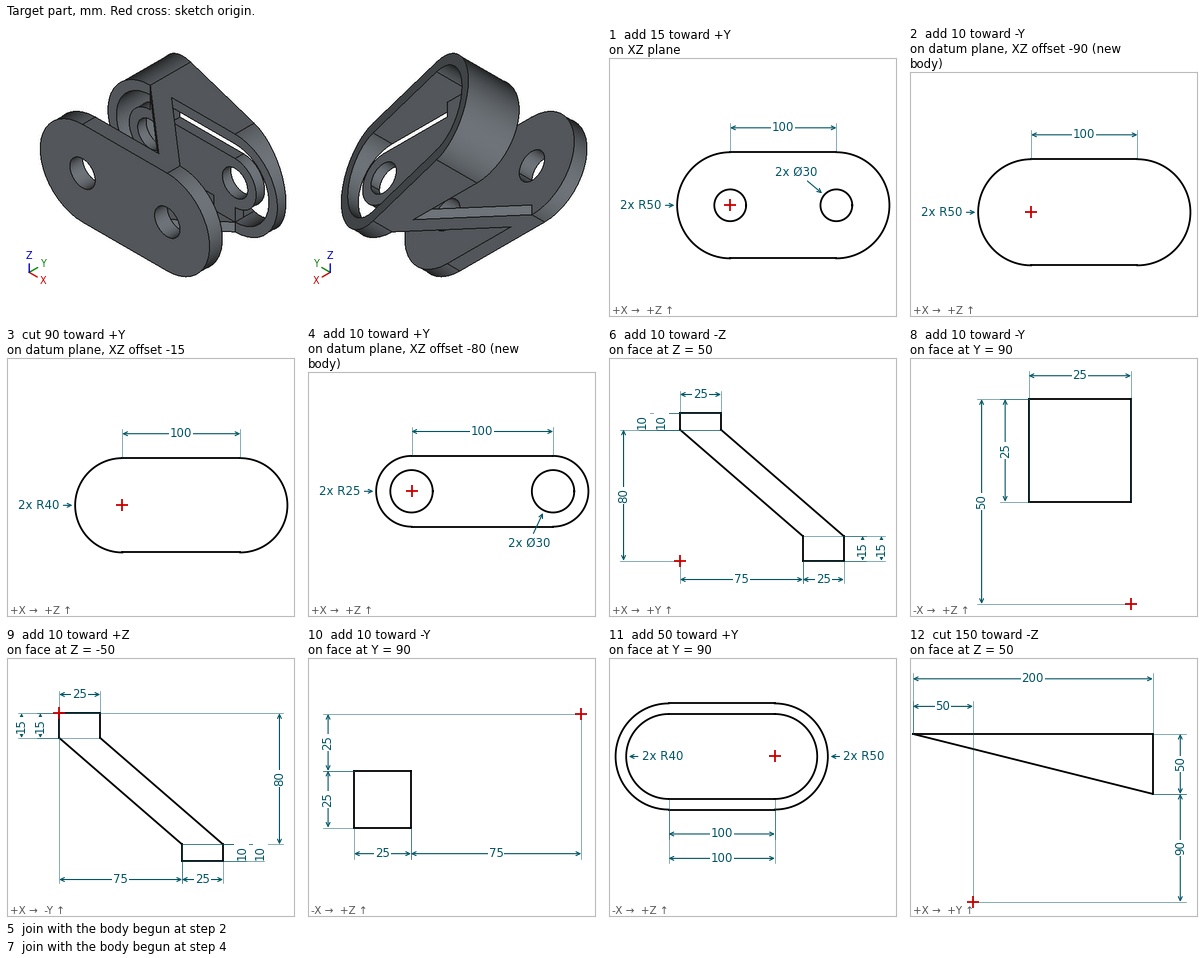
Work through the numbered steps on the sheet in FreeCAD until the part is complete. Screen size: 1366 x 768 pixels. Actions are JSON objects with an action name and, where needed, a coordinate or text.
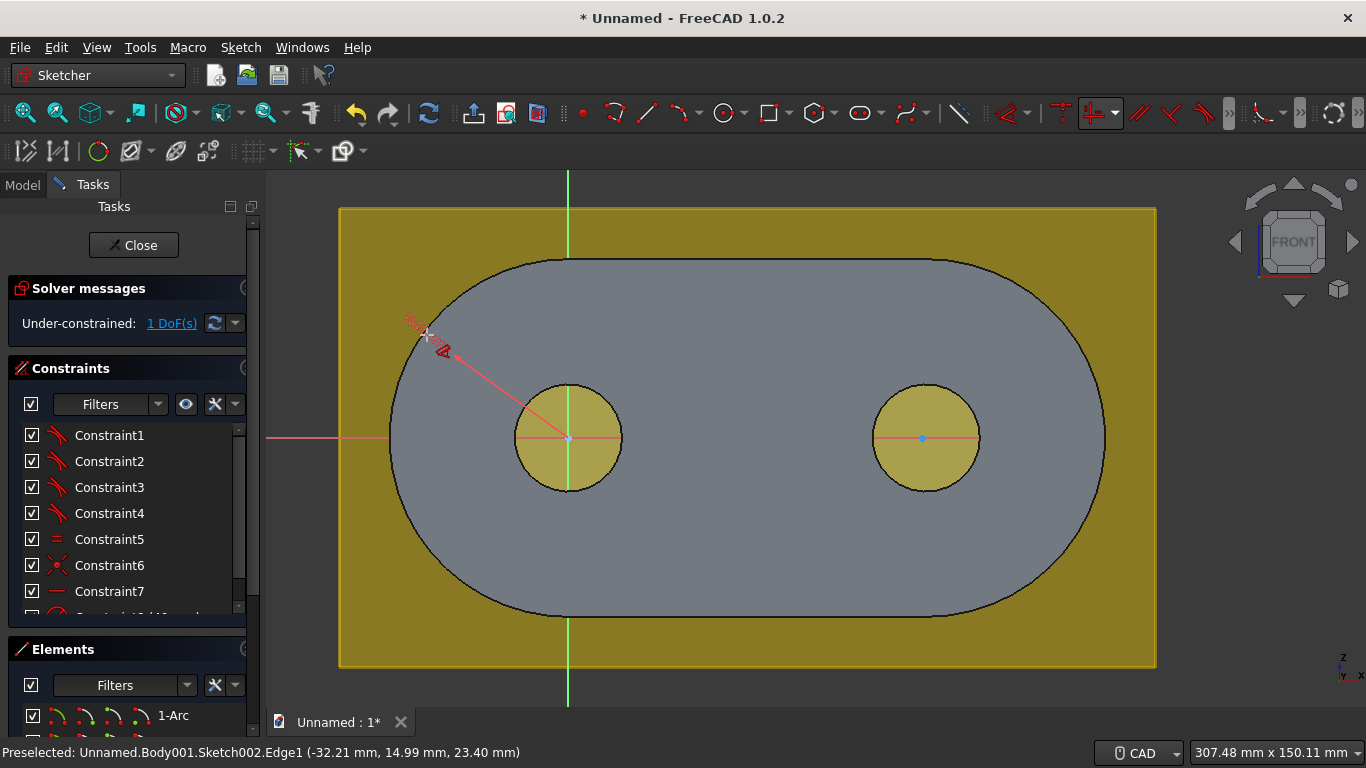
{"action": "left_click", "coordinate": [675, 295]}
{"action": "left_click", "coordinate": [746, 261]}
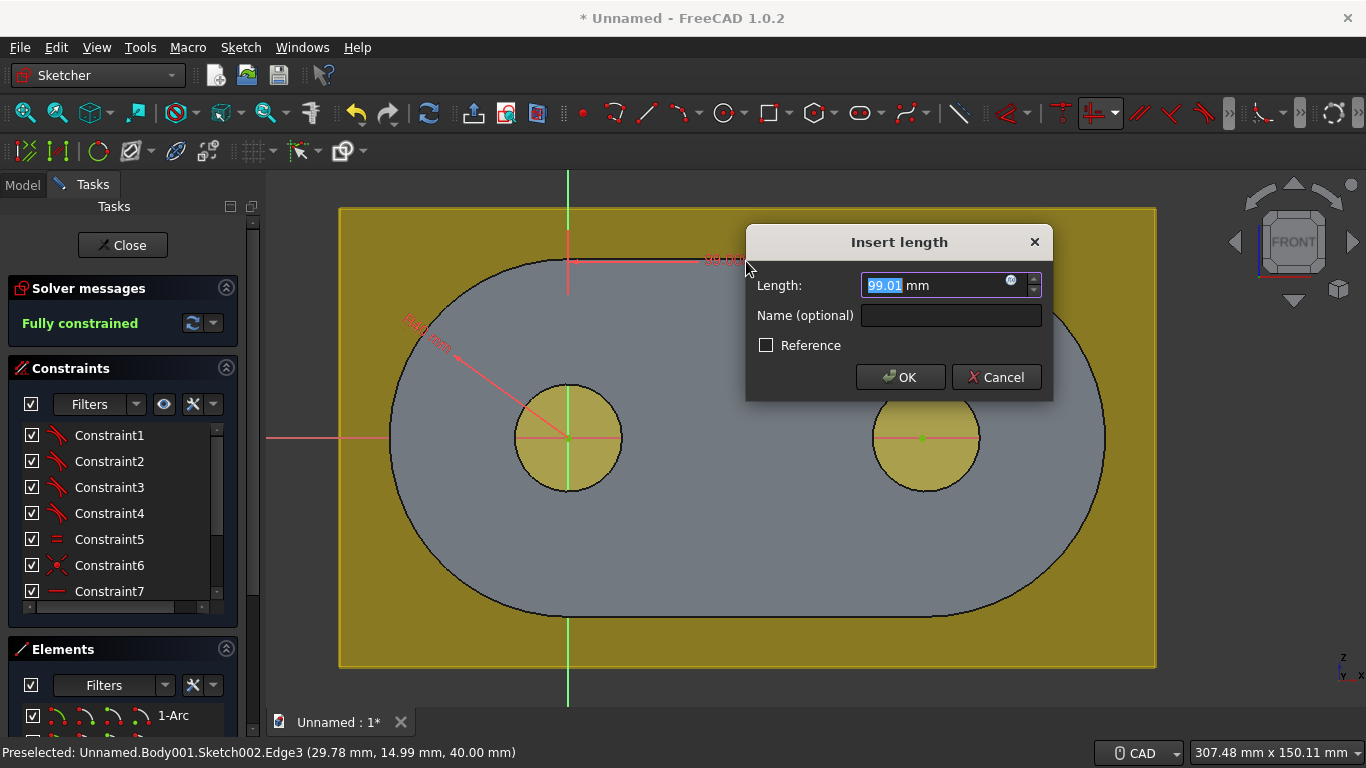
{"action": "type", "text": "100"}
{"action": "key", "text": "Return"}
{"action": "key", "text": "Escape"}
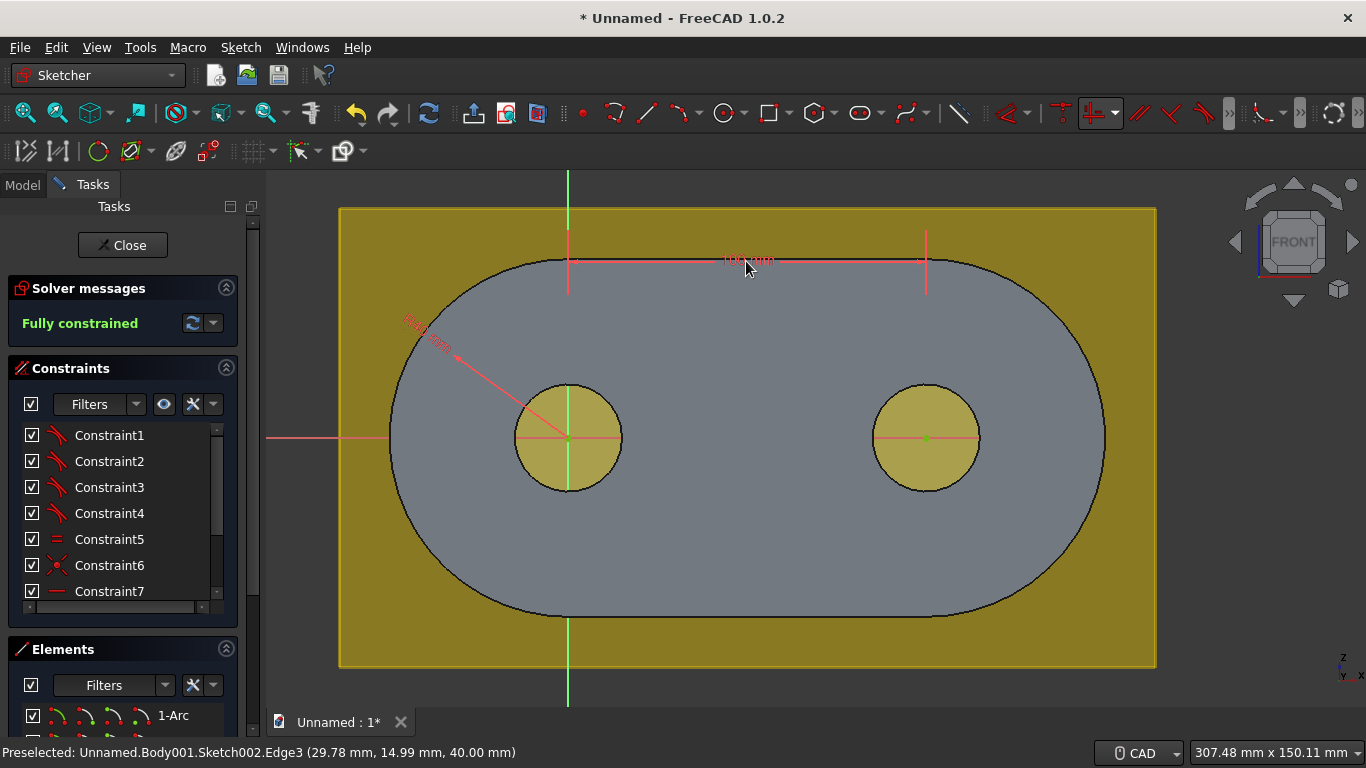
{"action": "left_click", "coordinate": [123, 245]}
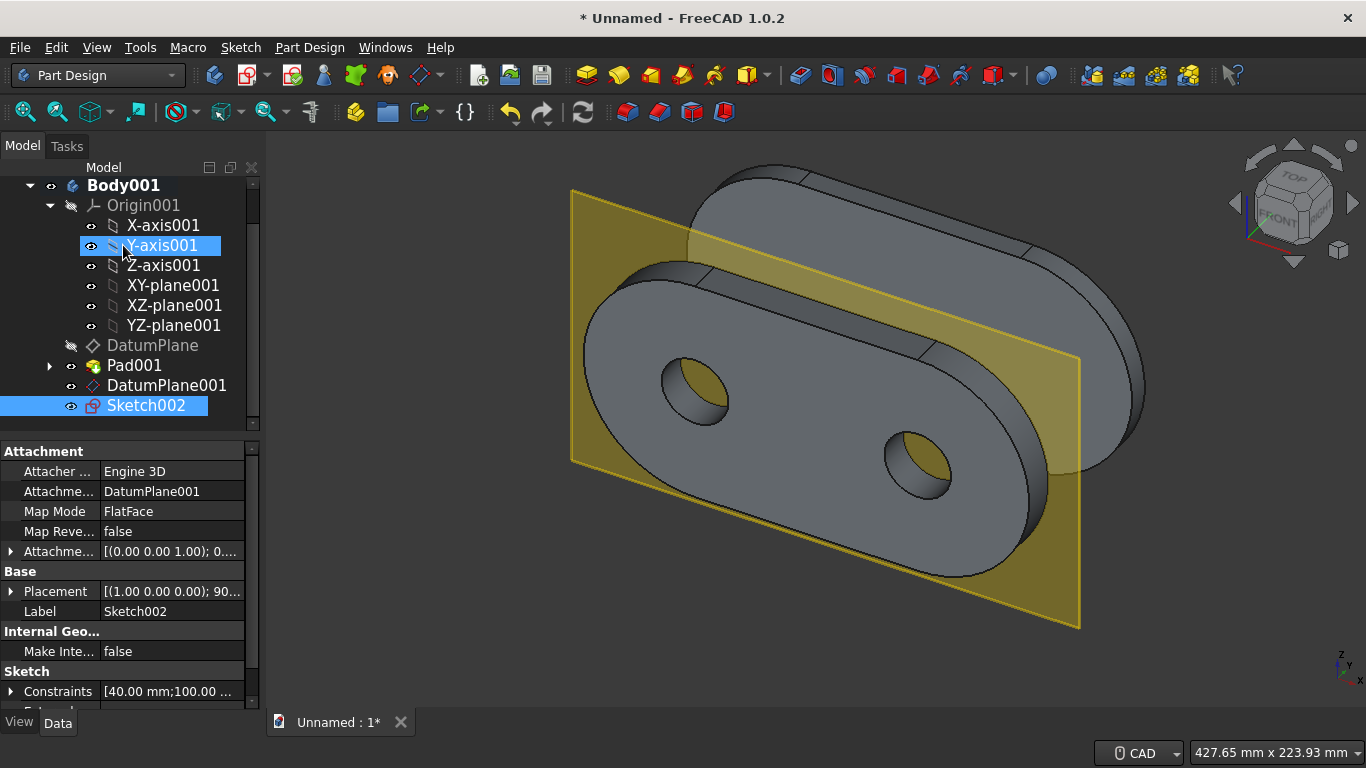
{"action": "left_click", "coordinate": [802, 76]}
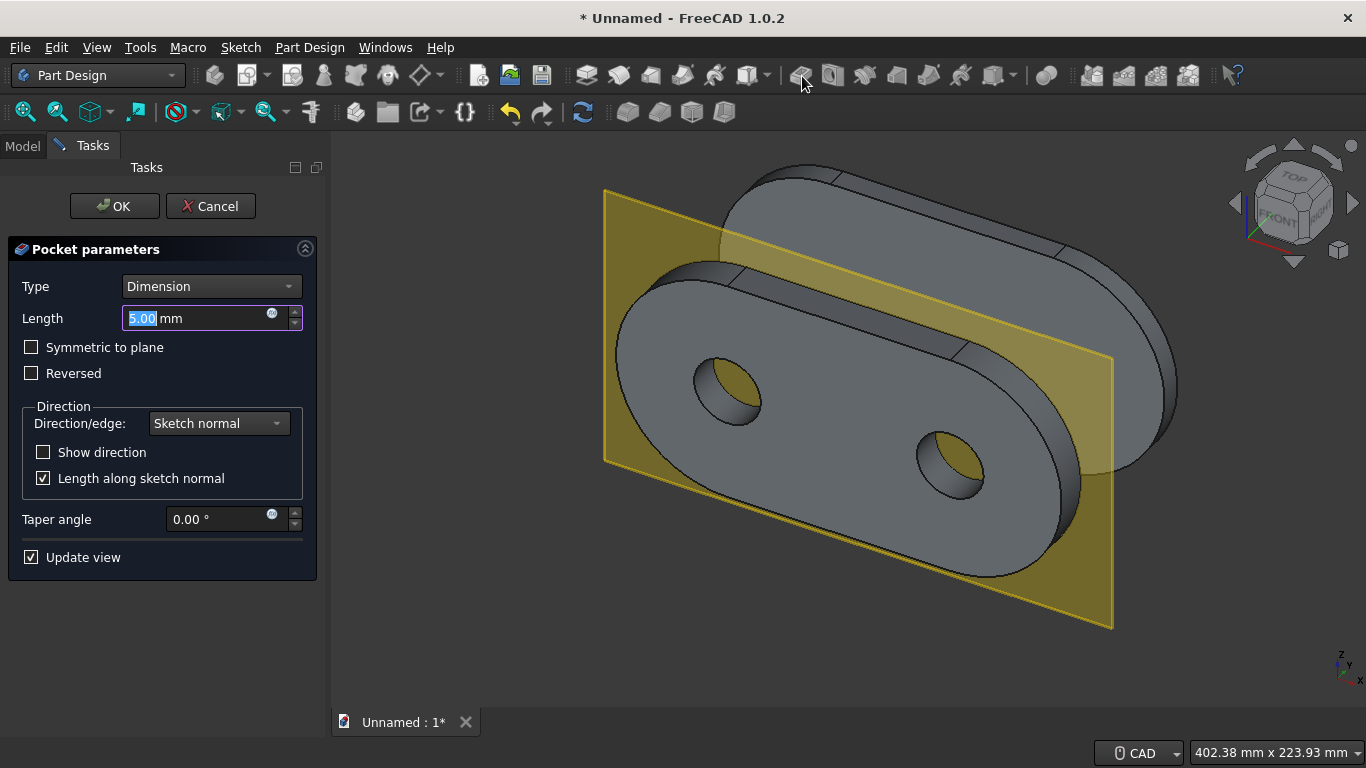
{"action": "type", "text": "90"}
{"action": "key", "text": "Tab"}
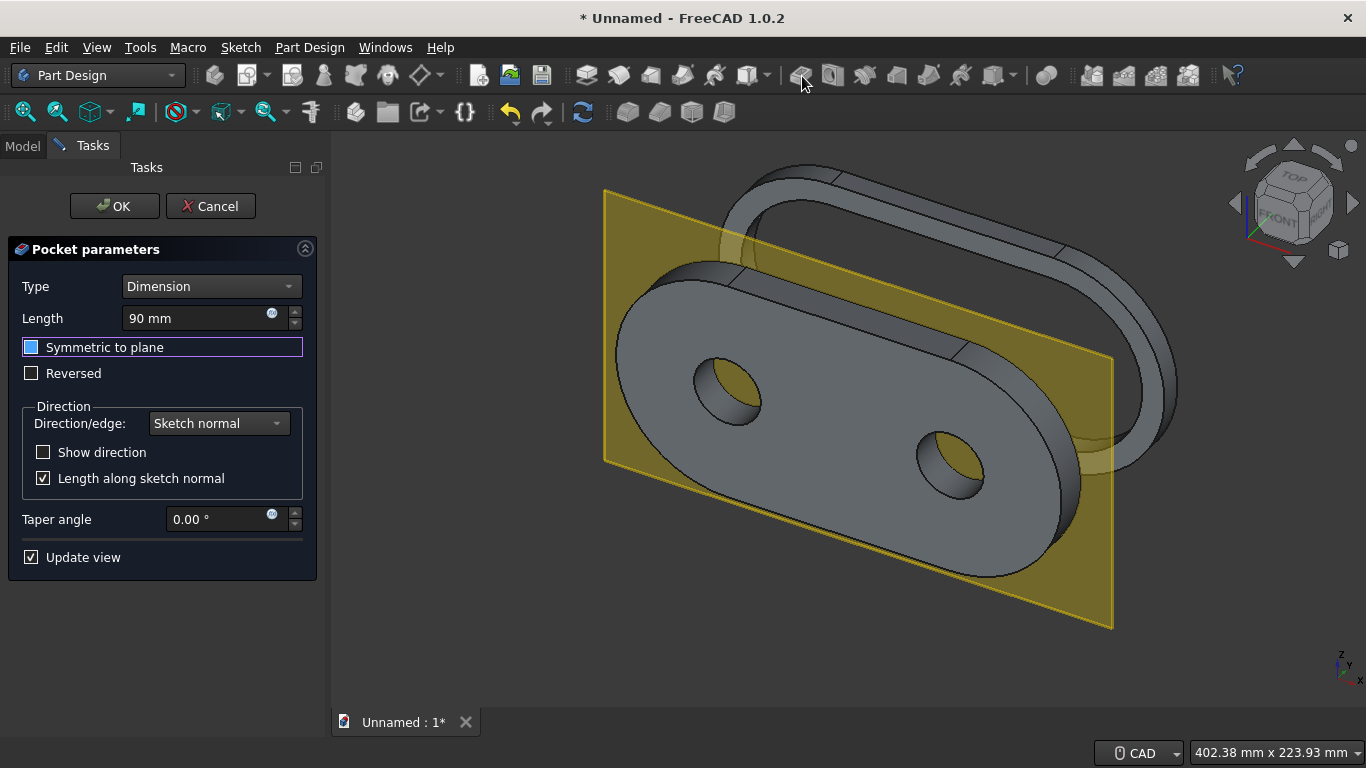
{"action": "left_click", "coordinate": [115, 206]}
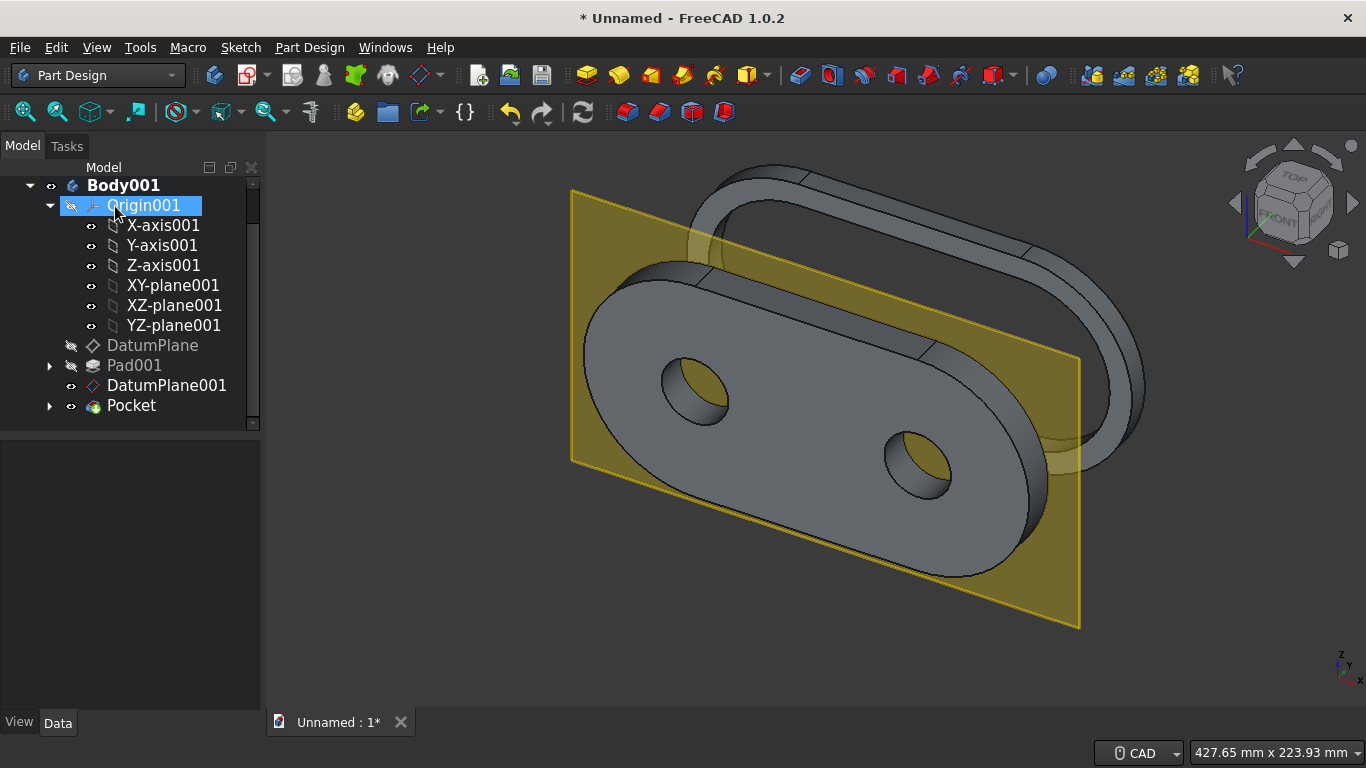
{"action": "left_click", "coordinate": [116, 386]}
{"action": "key", "text": "space"}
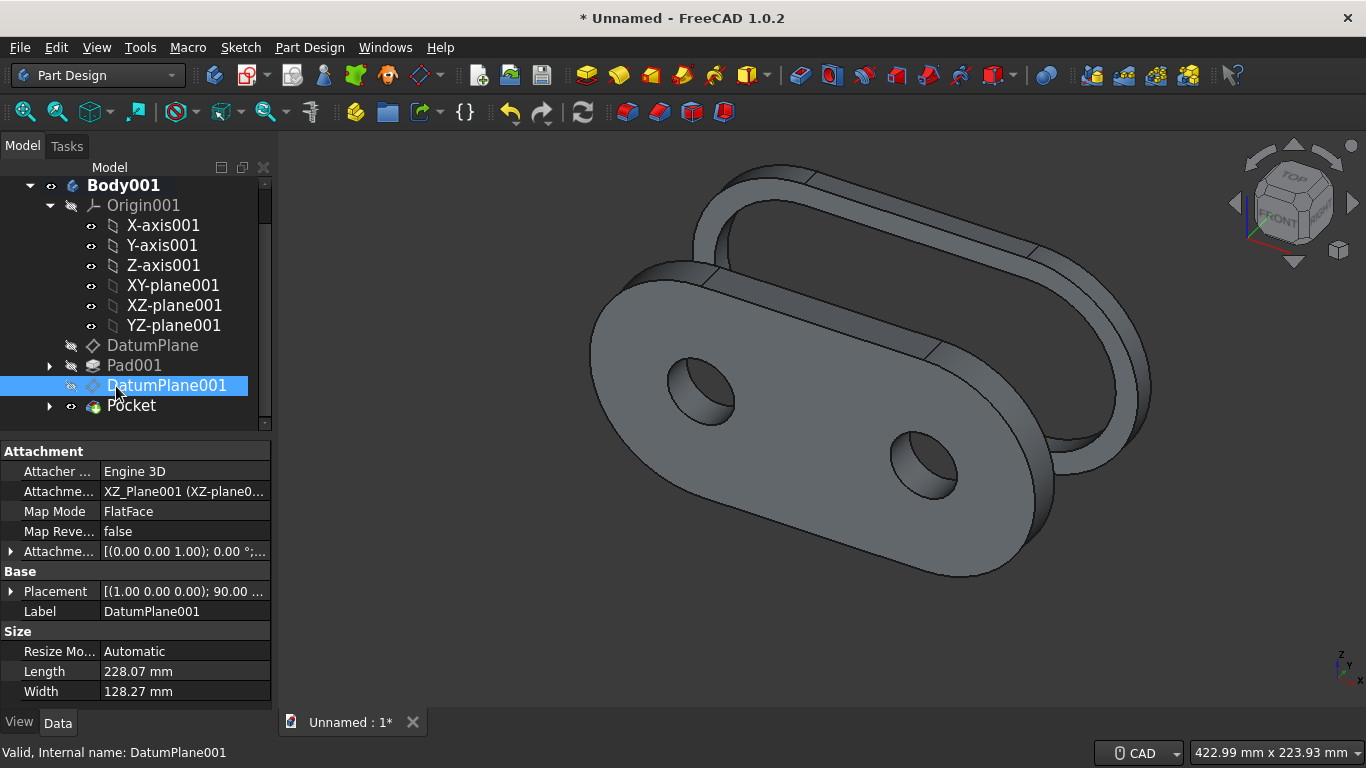
{"action": "left_click", "coordinate": [318, 667]}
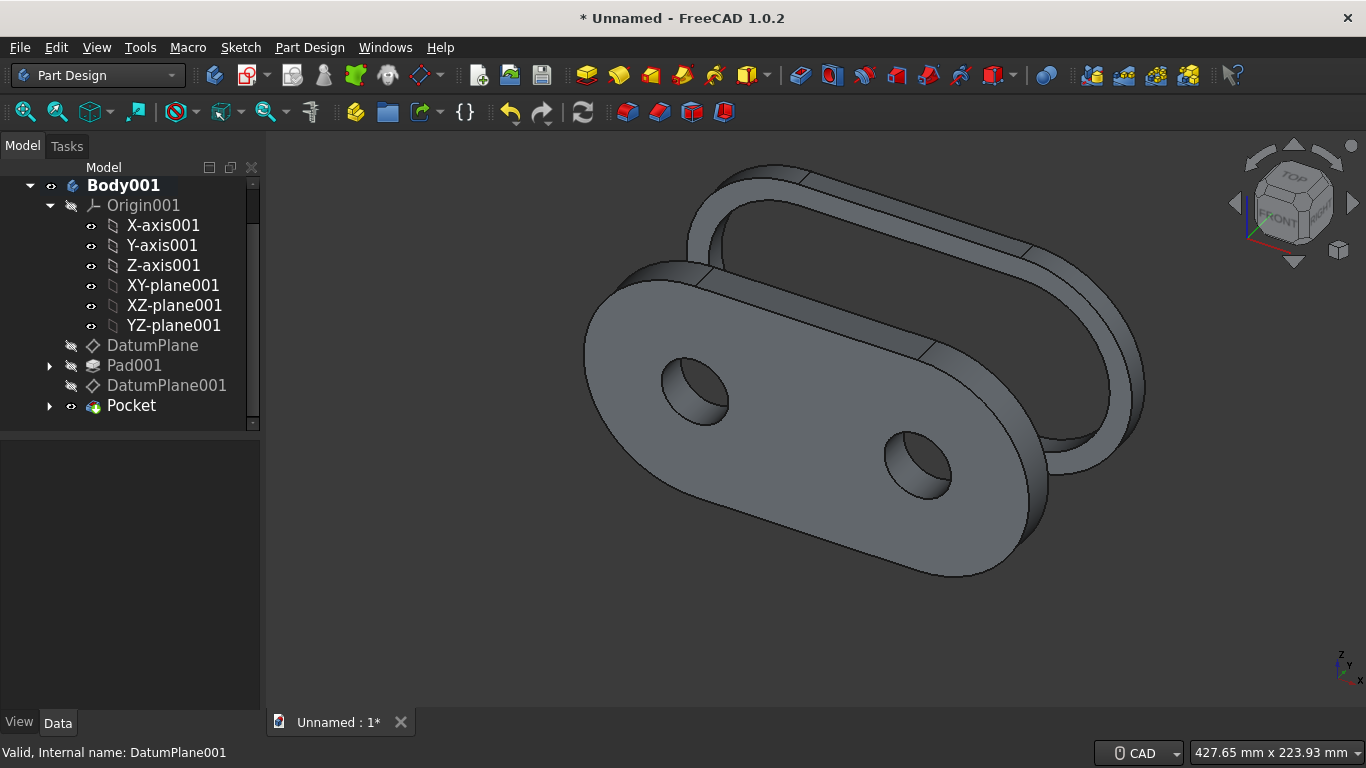
{"action": "left_click", "coordinate": [216, 76]}